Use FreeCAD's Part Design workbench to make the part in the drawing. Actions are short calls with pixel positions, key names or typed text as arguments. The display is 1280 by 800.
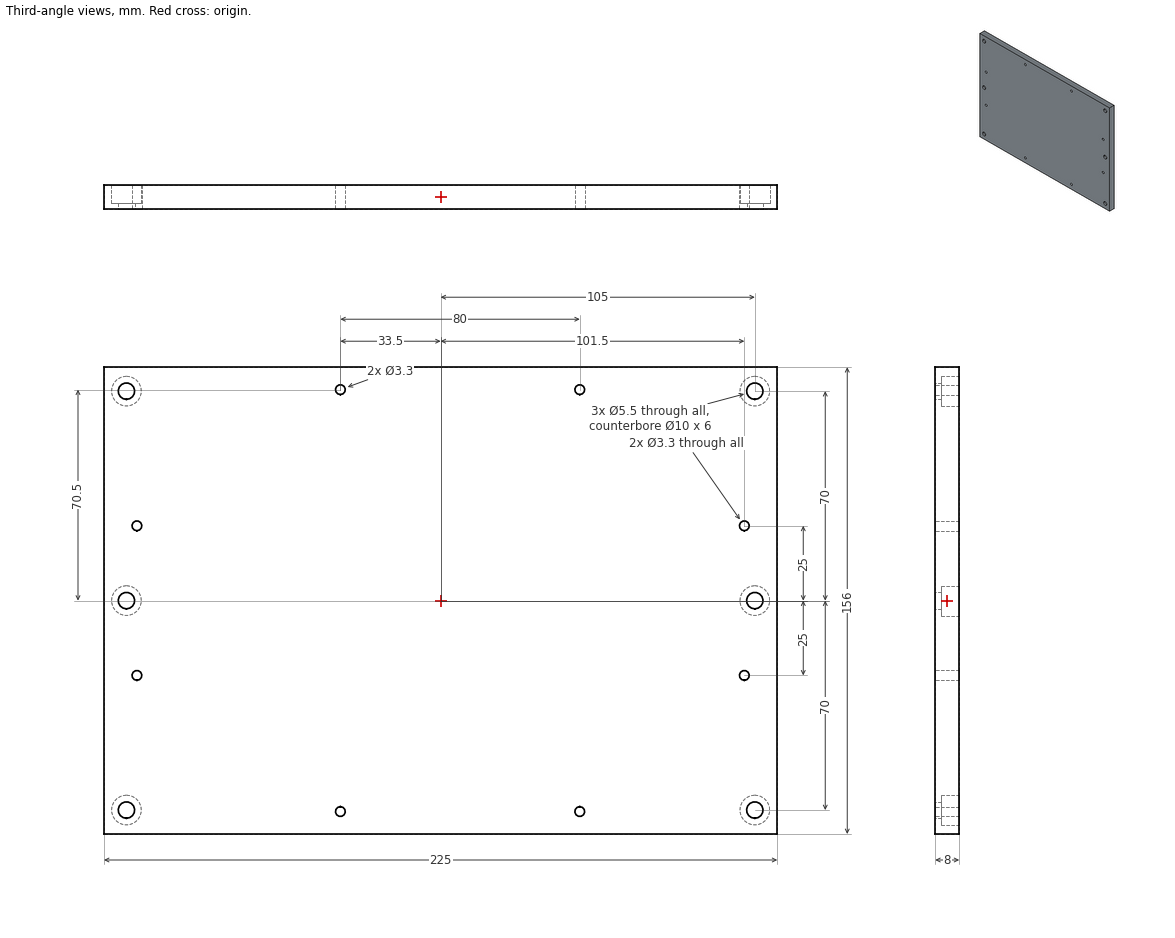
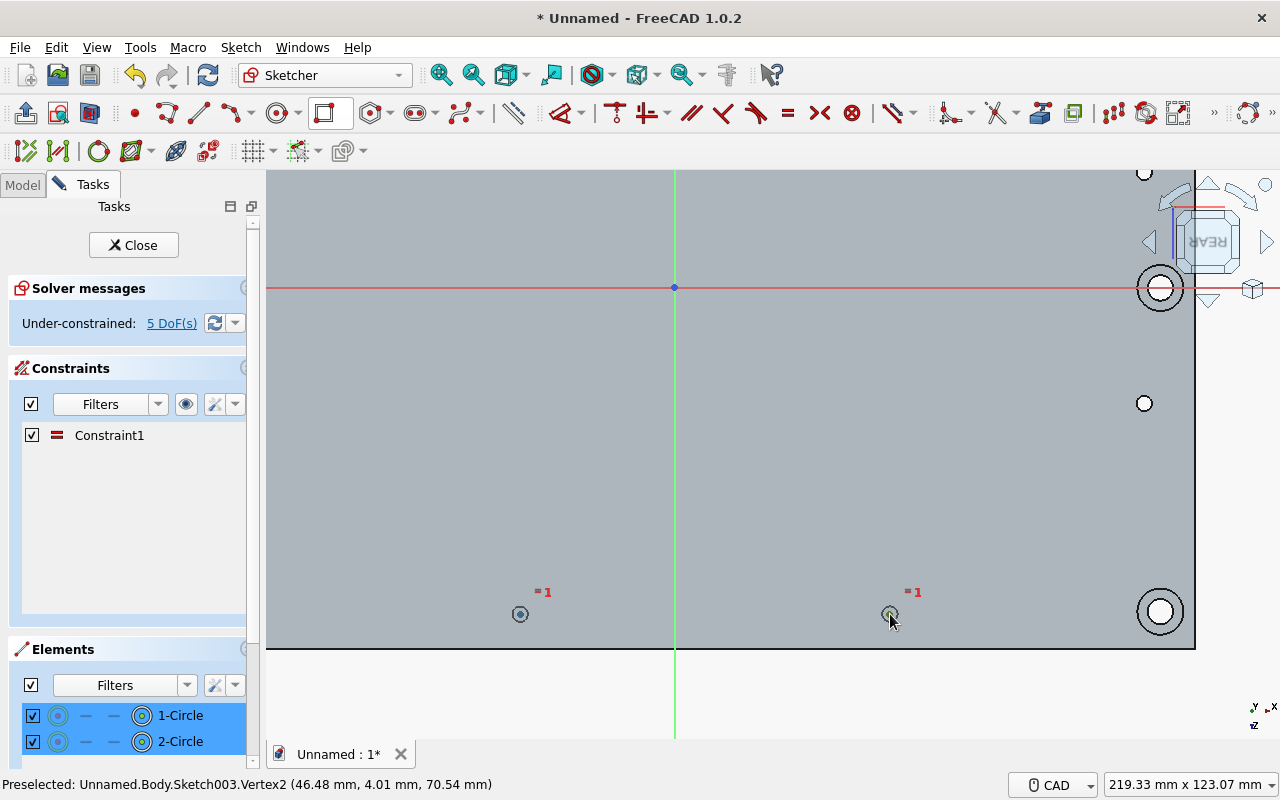
key(h)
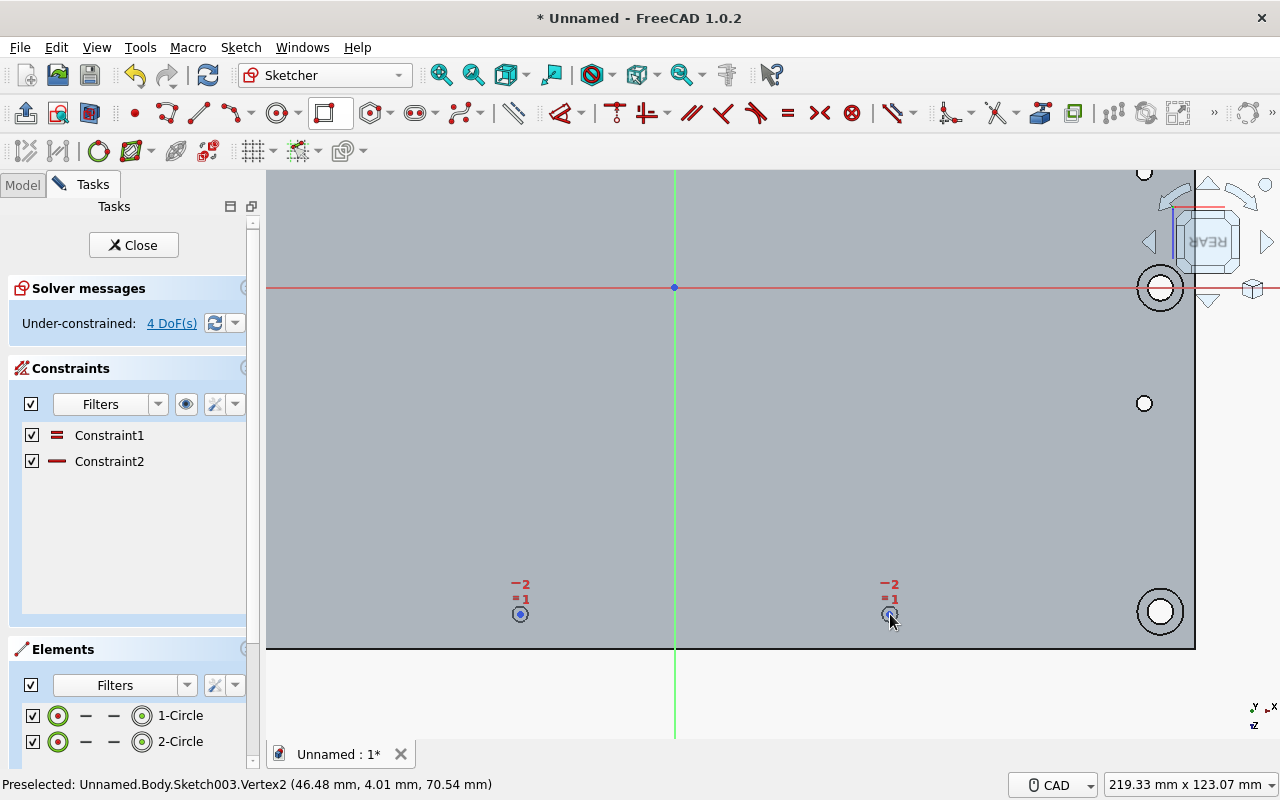
key(d)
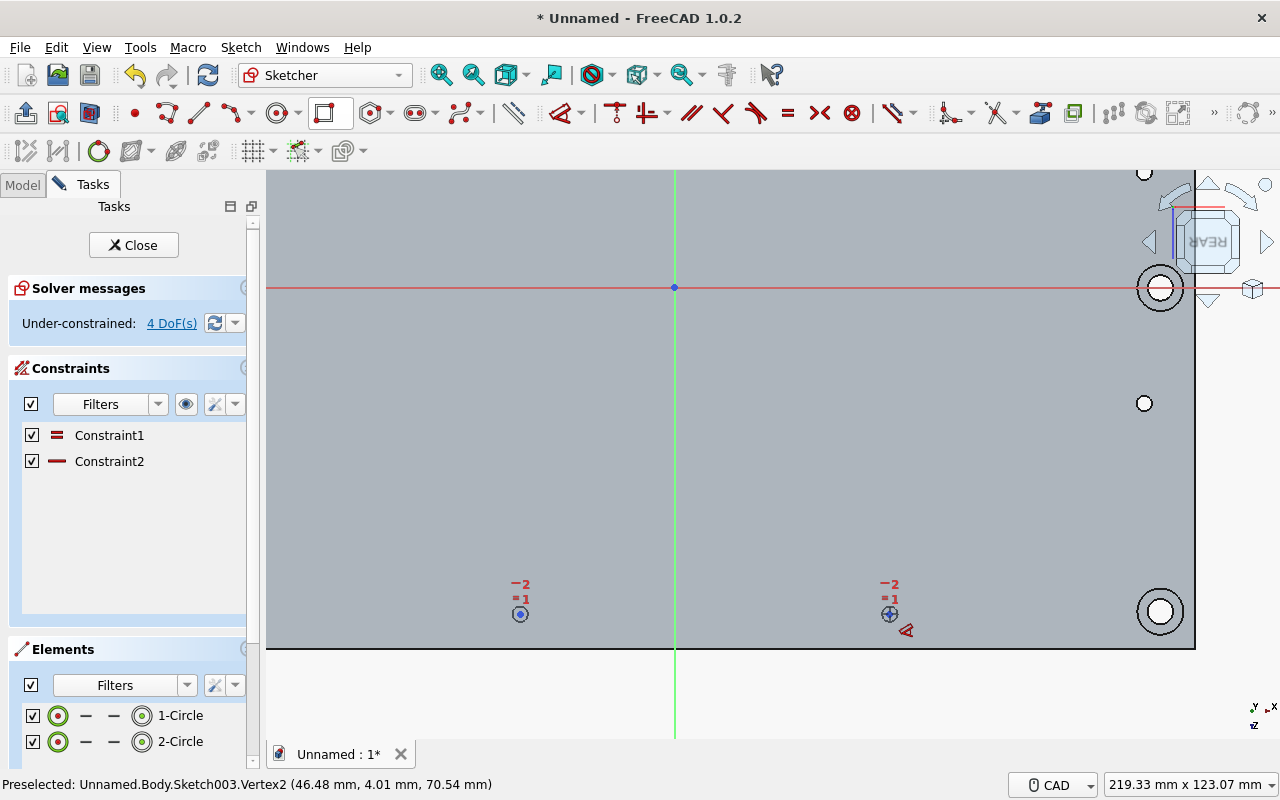
scroll(520, 607, up, 5)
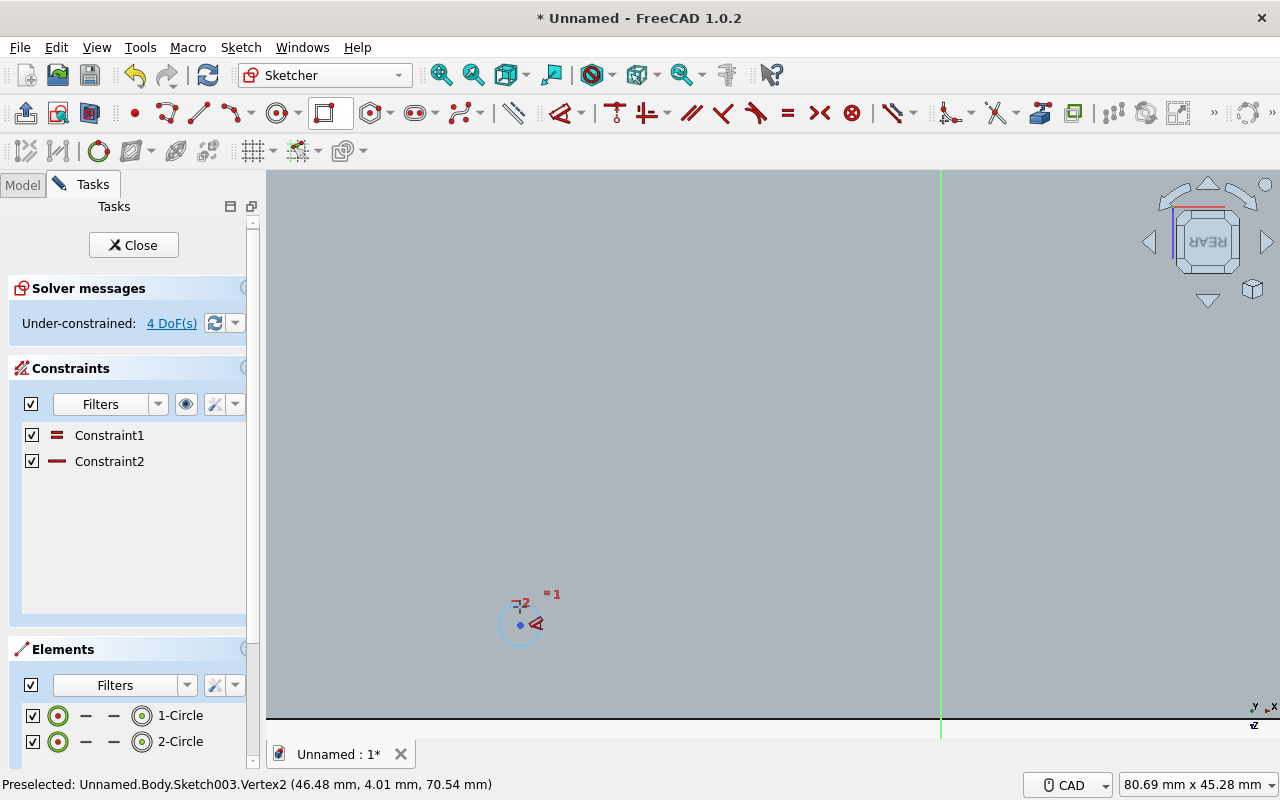
click(521, 604)
click(522, 572)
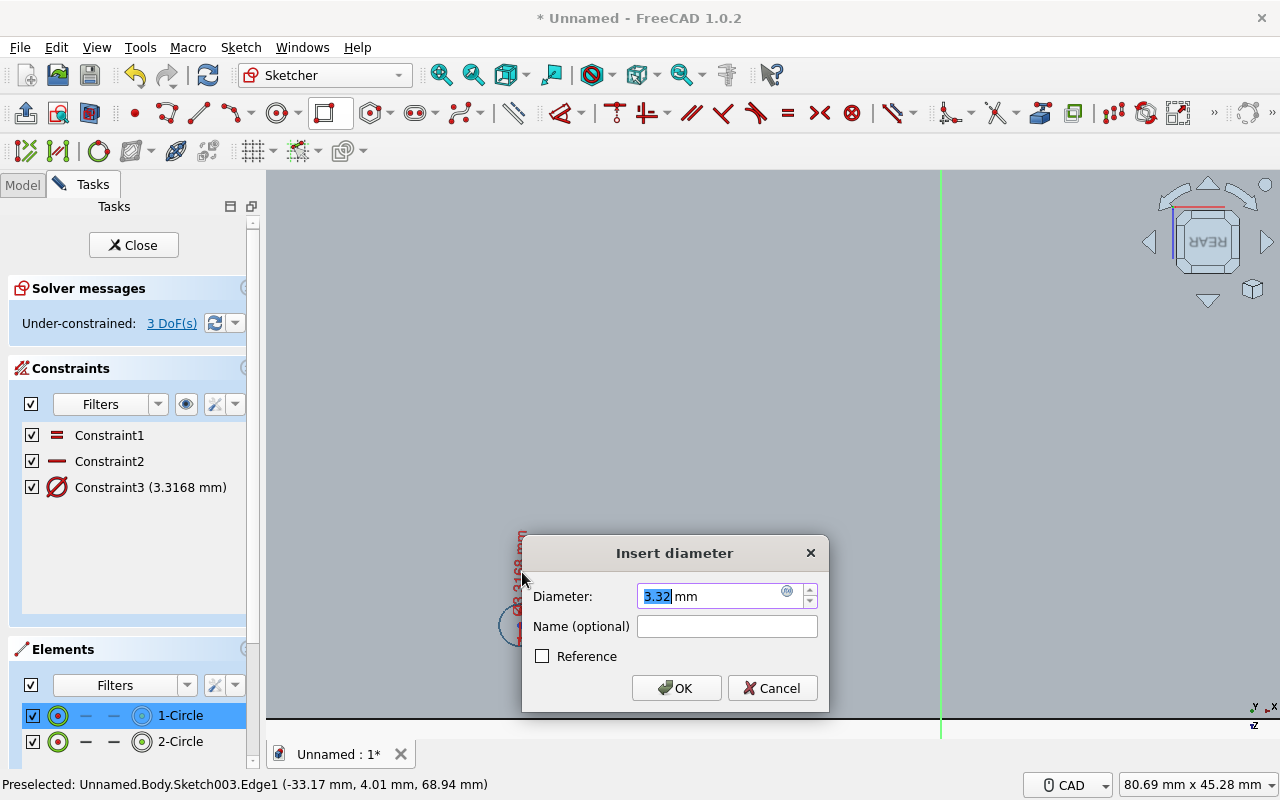
text(3.3)
key(Return)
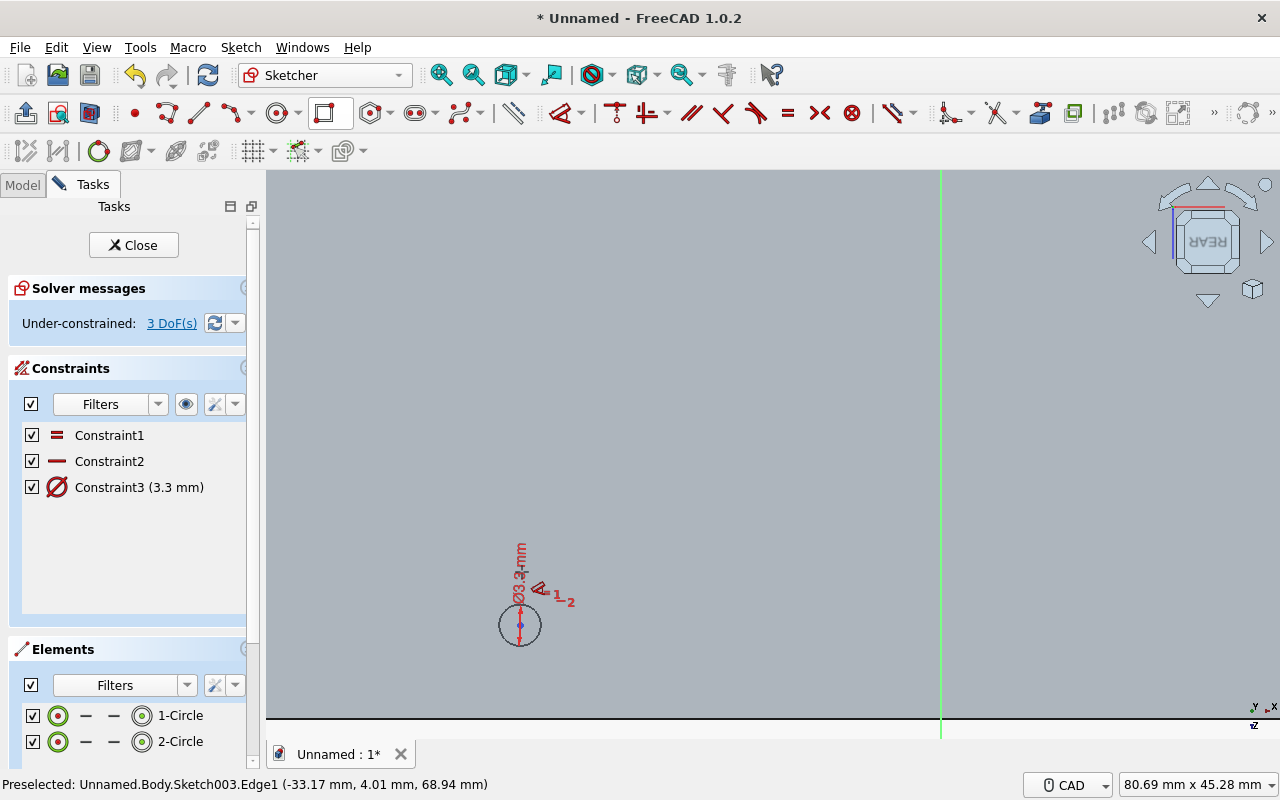
click(520, 625)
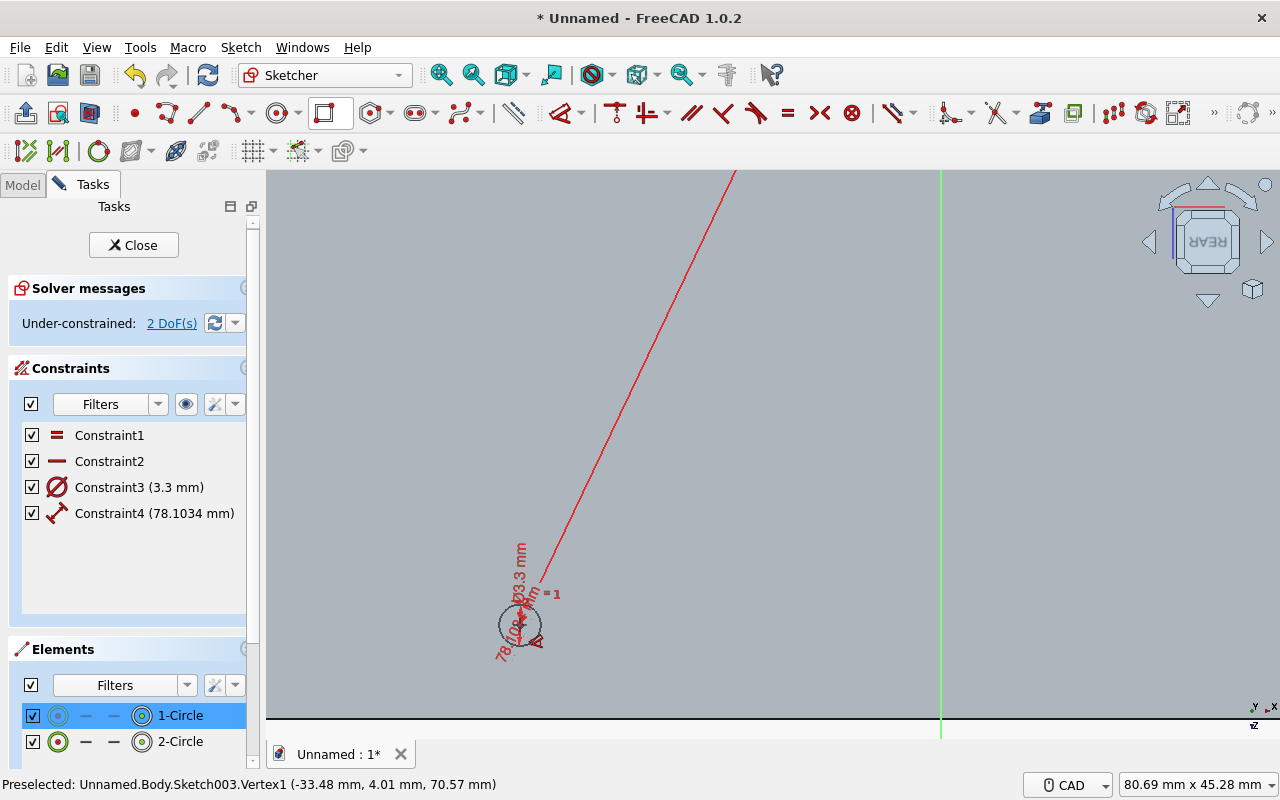
scroll(519, 607, down, 5)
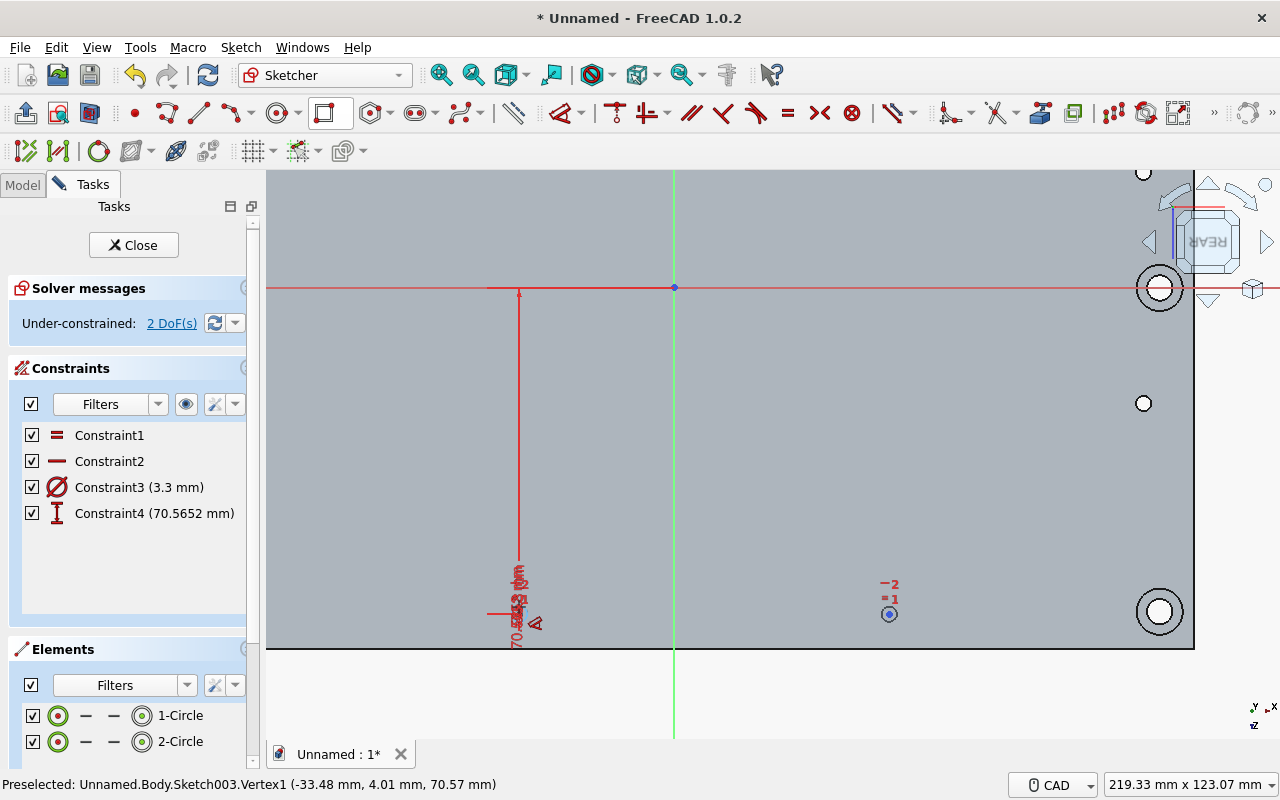
click(889, 614)
click(704, 648)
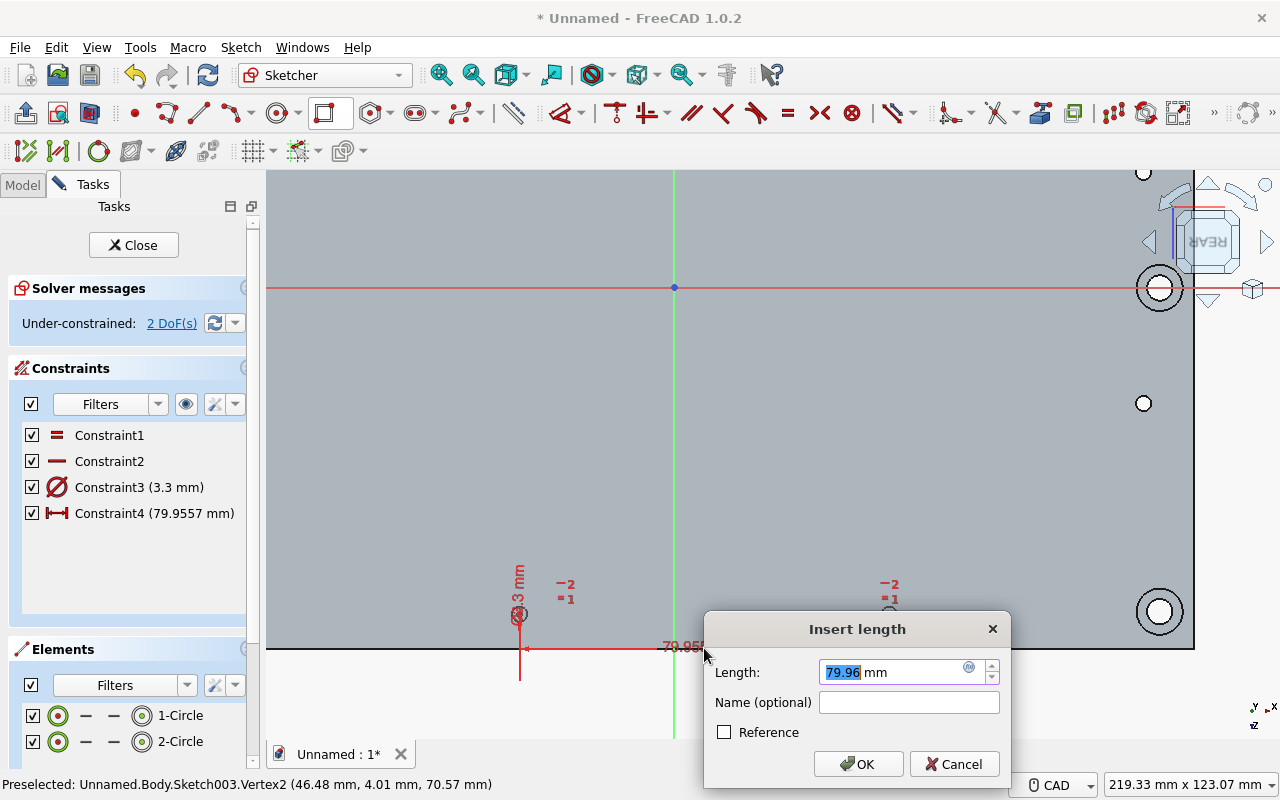
text(80)
key(Return)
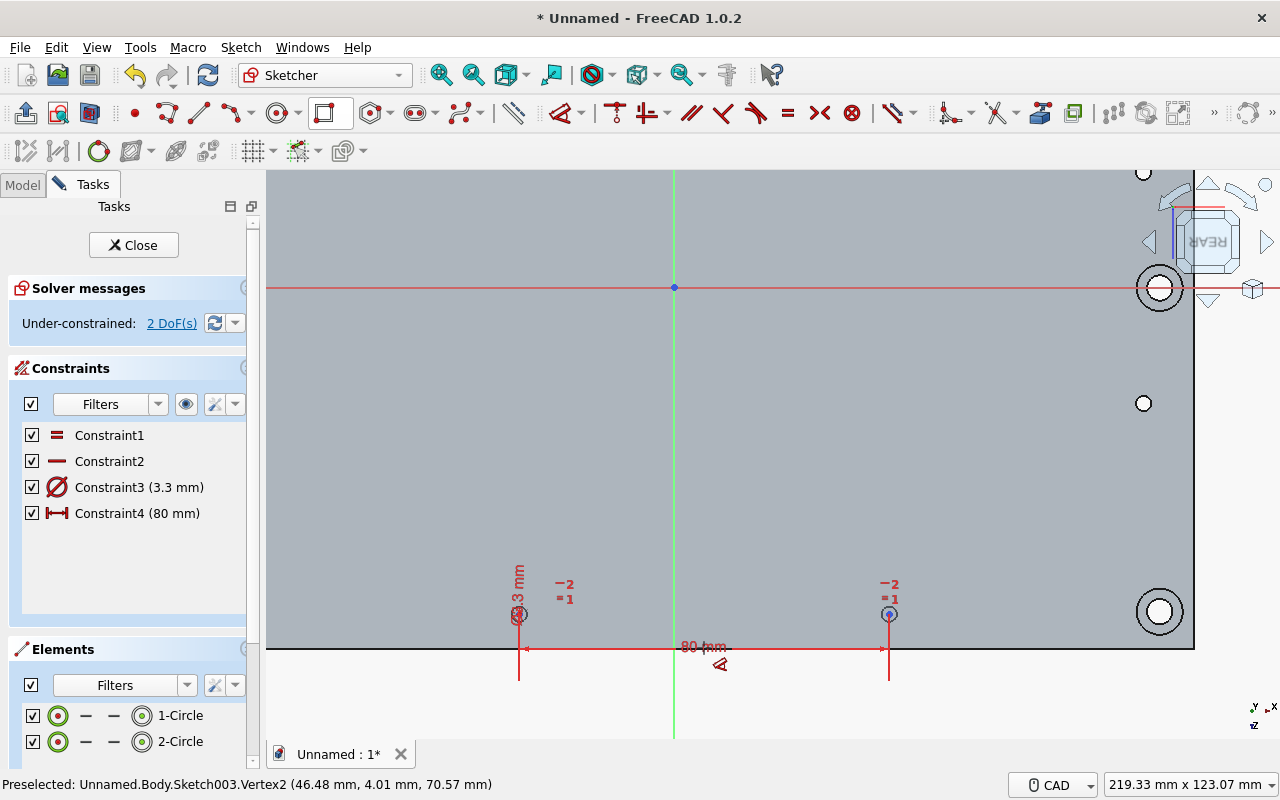
click(519, 614)
click(597, 254)